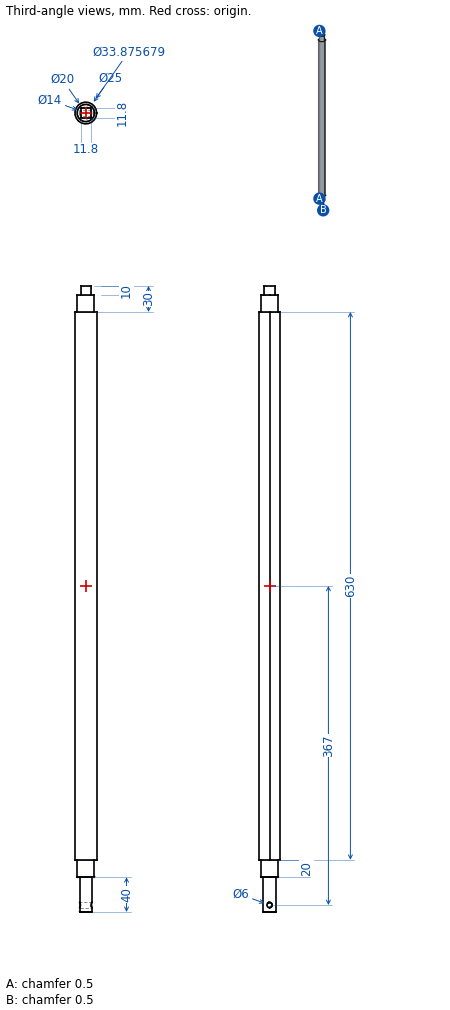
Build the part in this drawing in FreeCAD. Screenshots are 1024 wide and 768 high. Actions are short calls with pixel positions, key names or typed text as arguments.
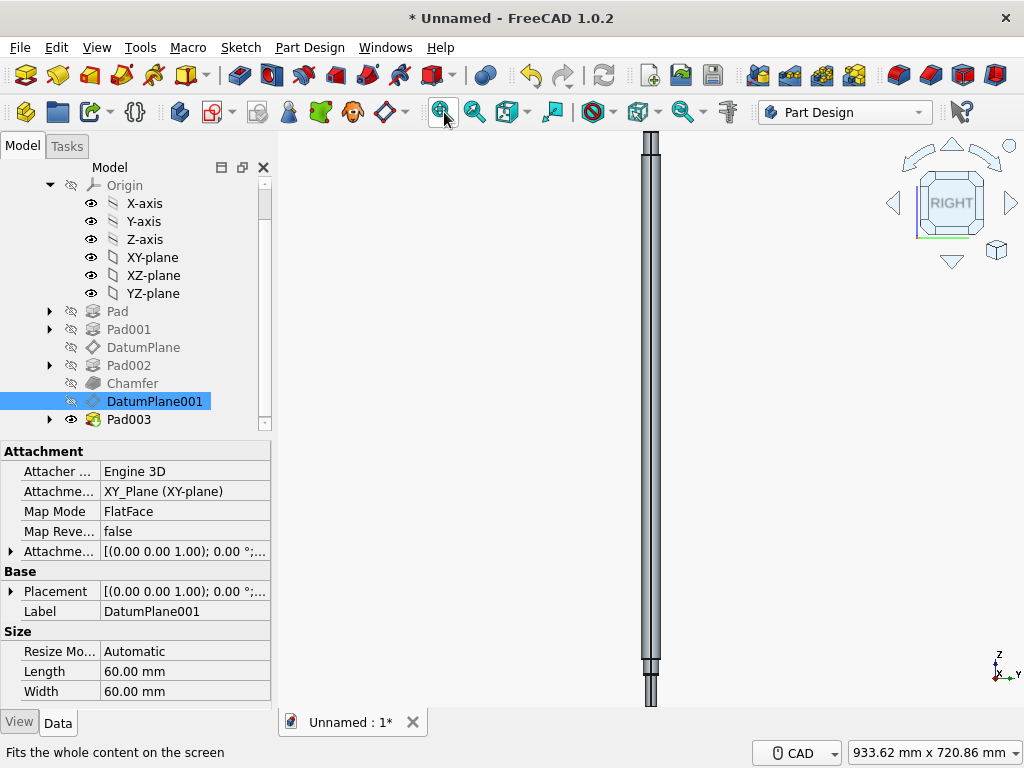
key(0)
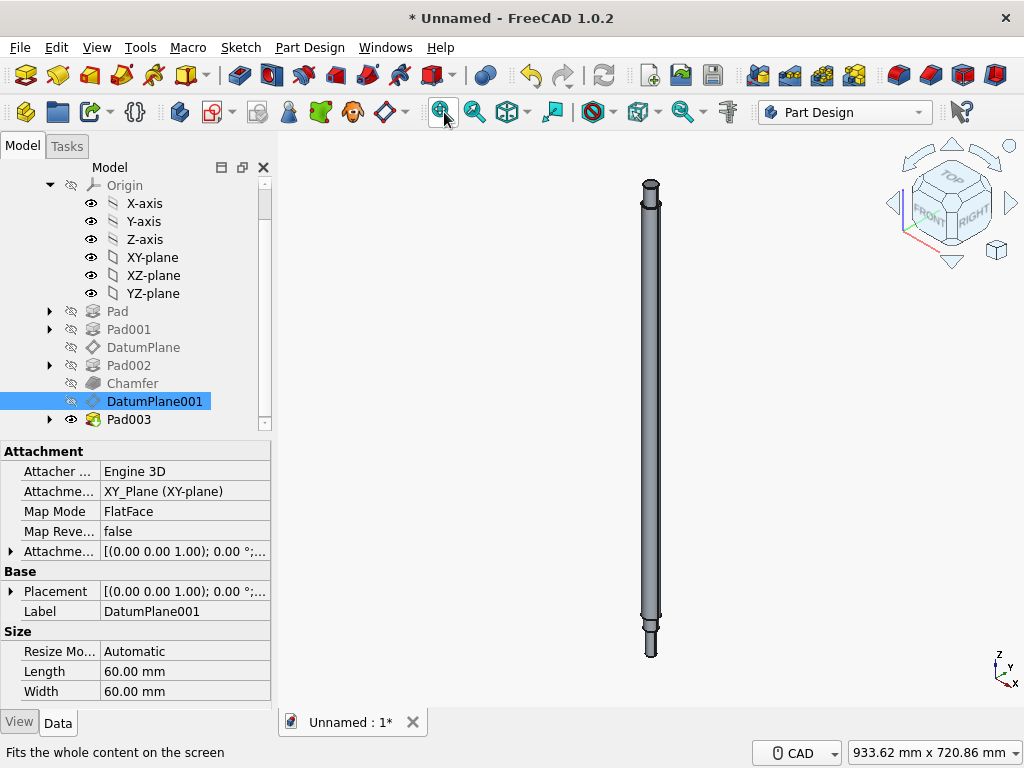
click(656, 655)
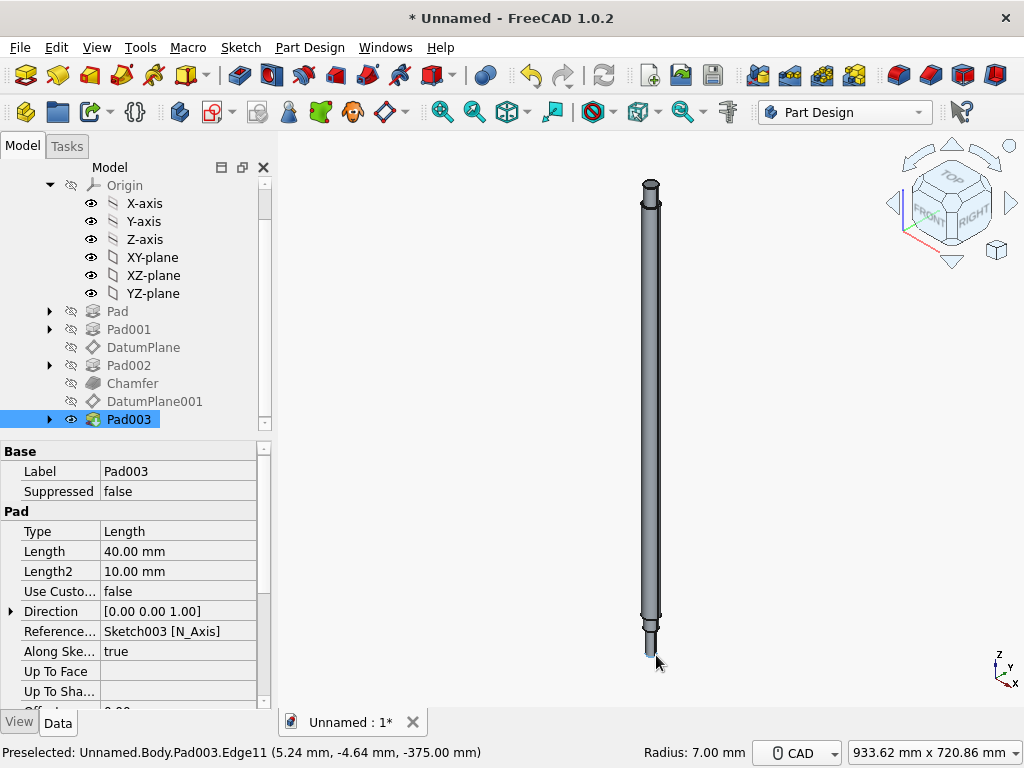
click(932, 76)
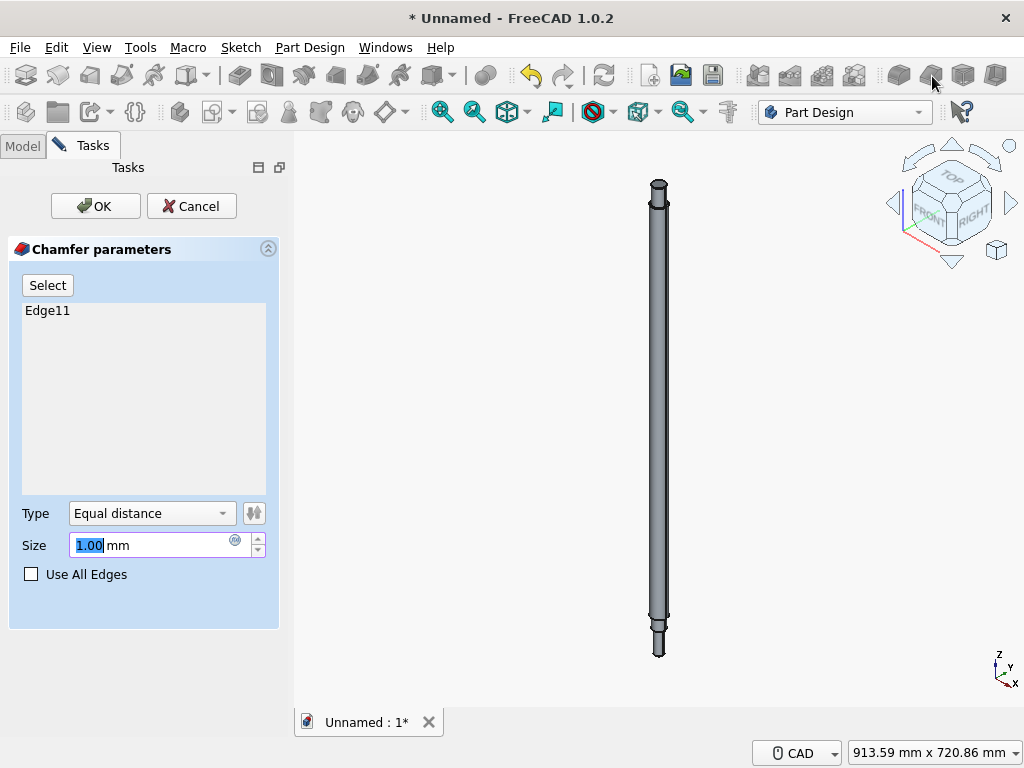
text(0.5)
key(Tab)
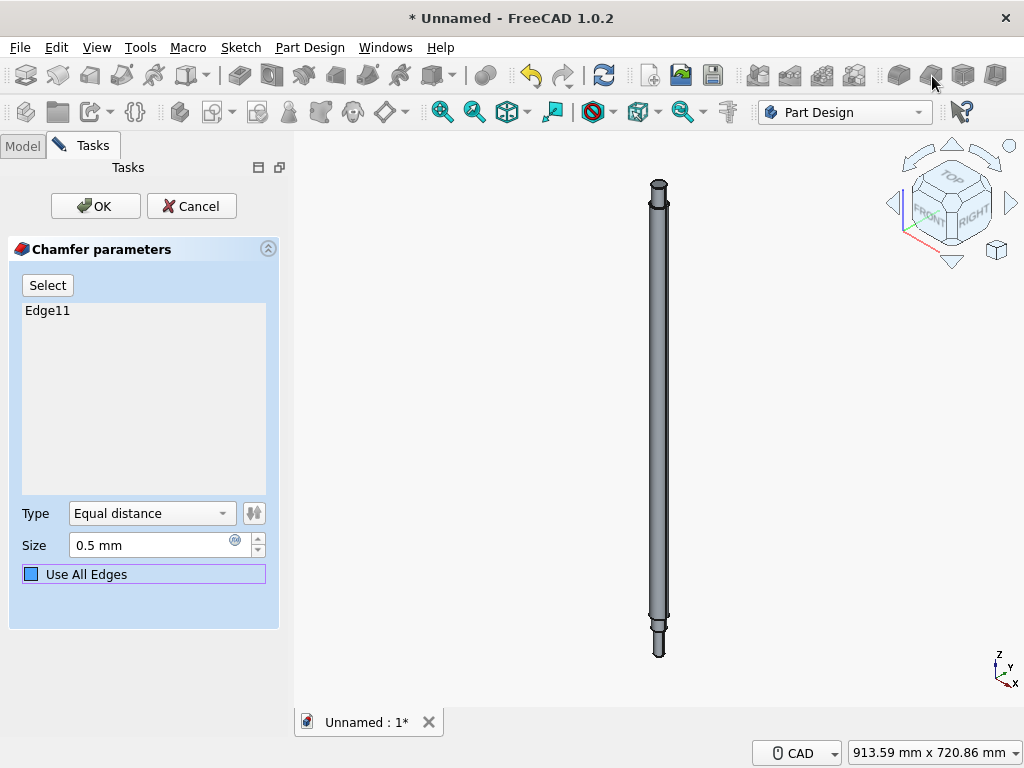
click(96, 206)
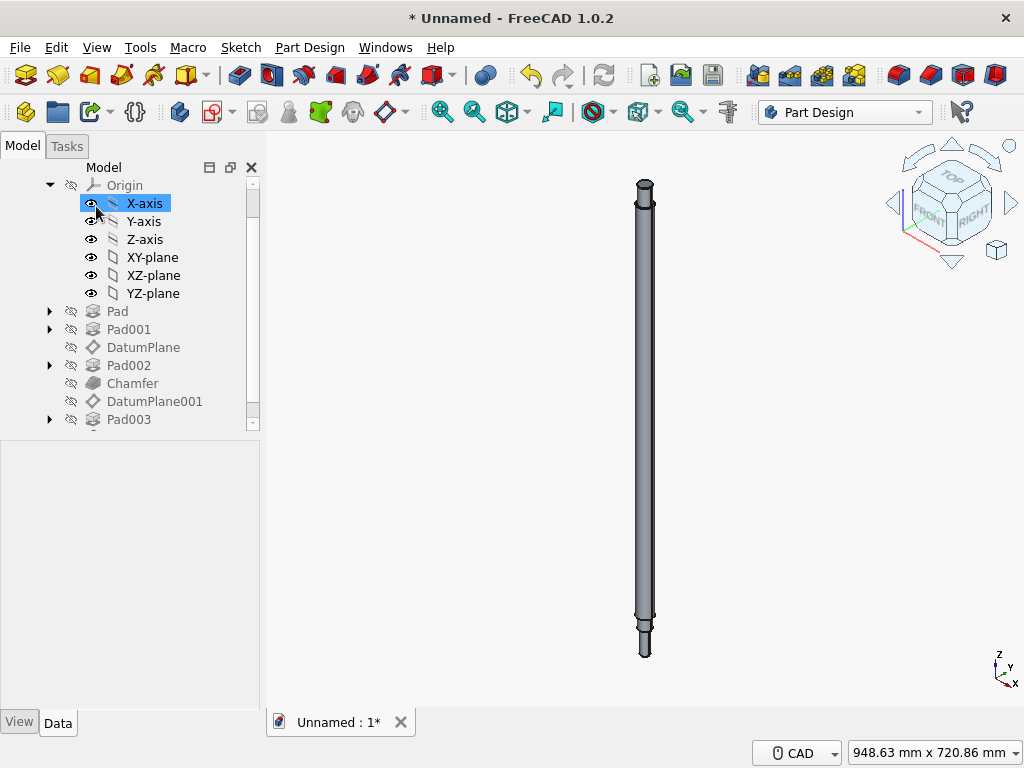
click(212, 112)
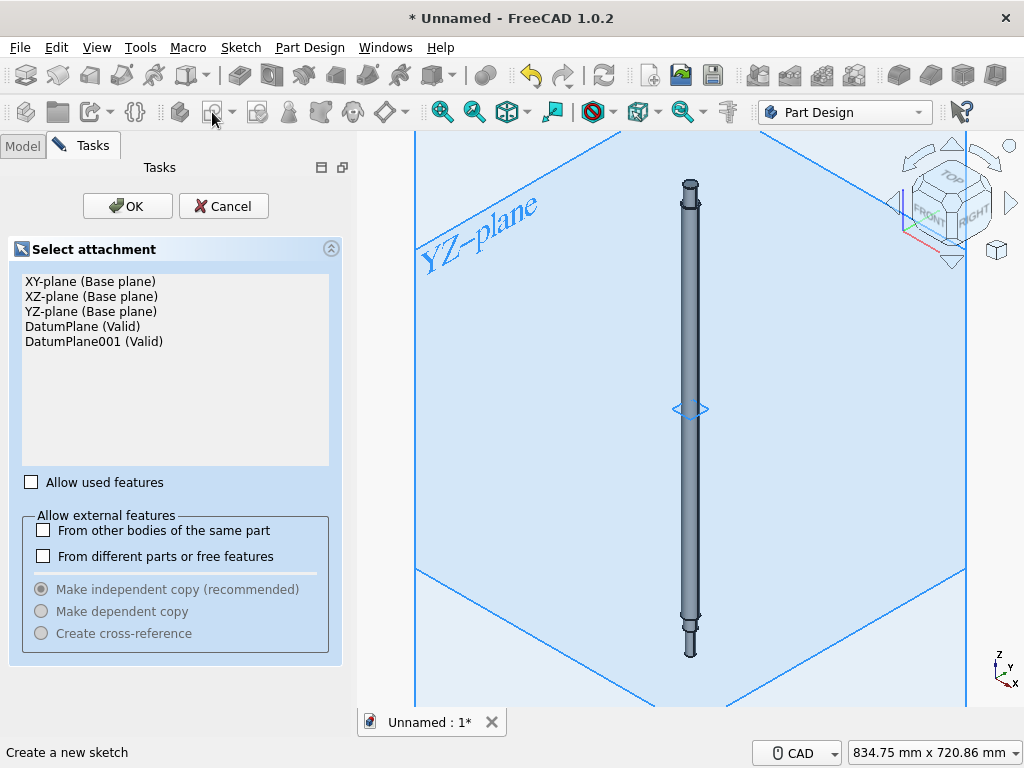
click(82, 312)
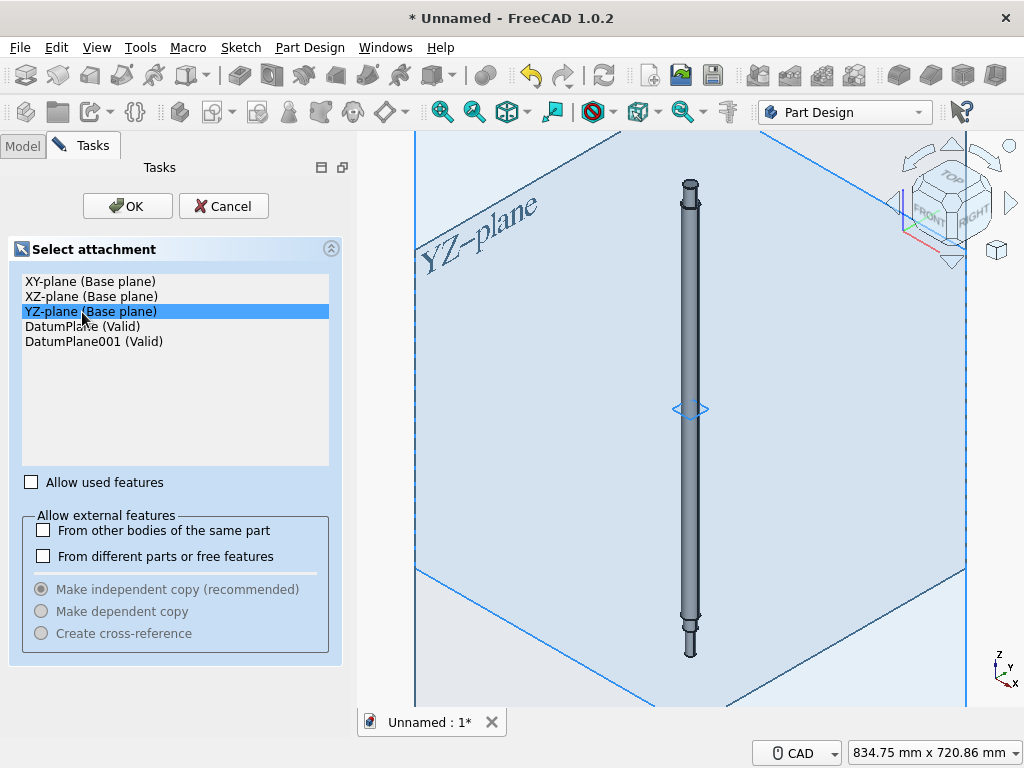
click(128, 206)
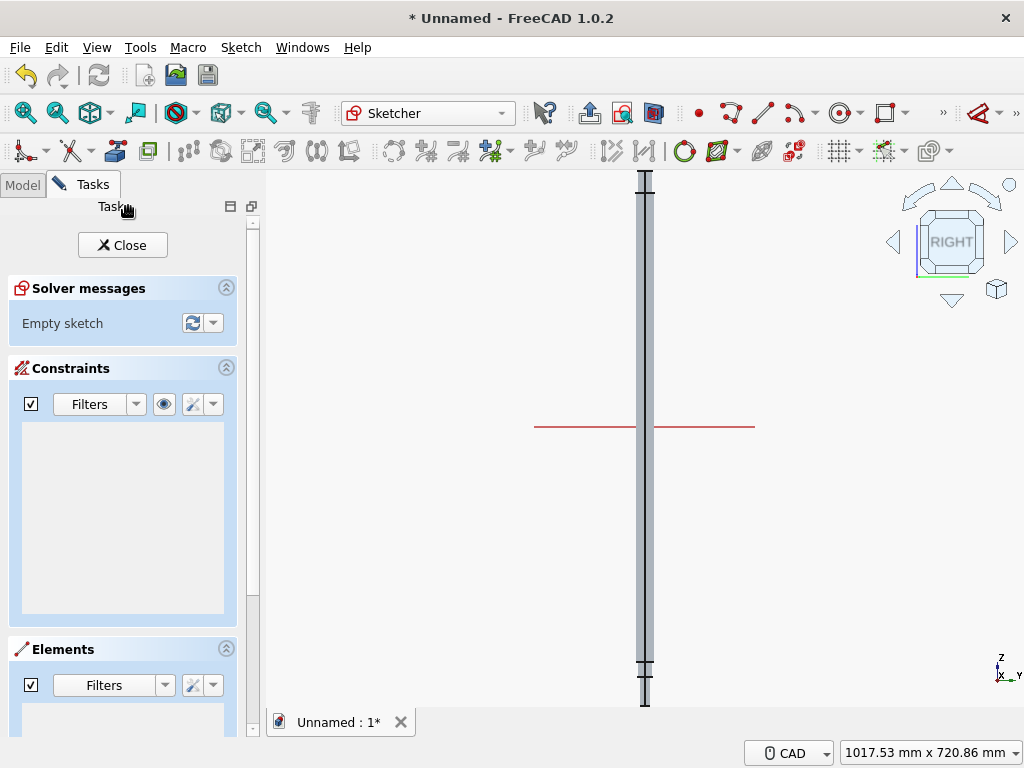
click(654, 114)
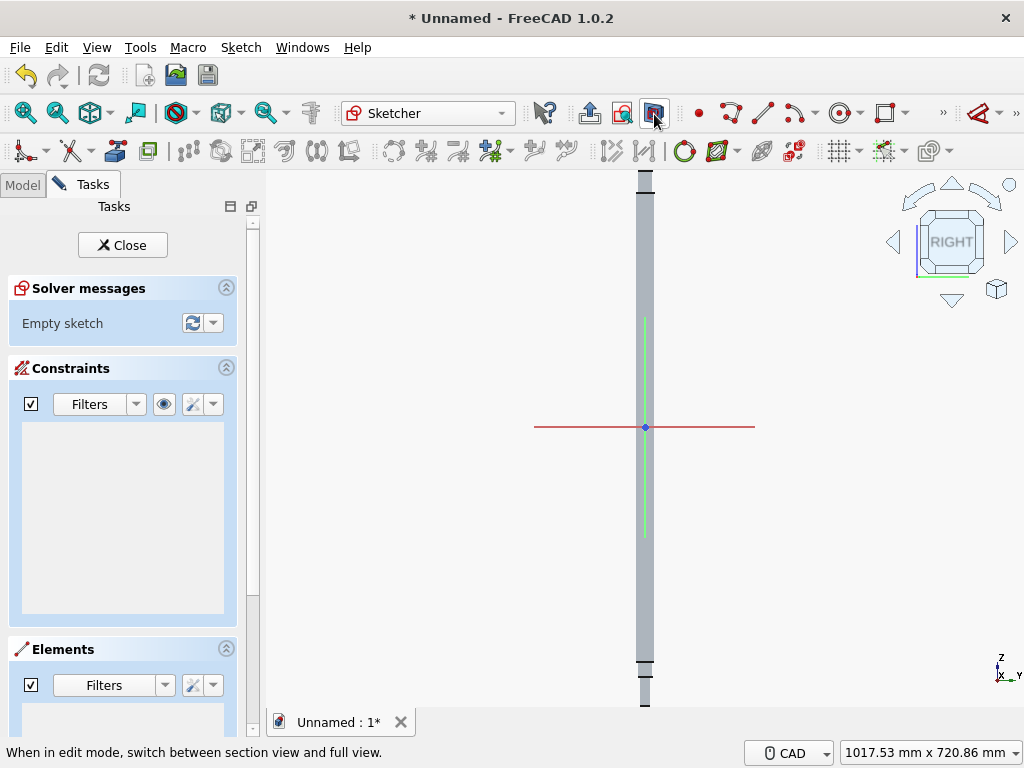
scroll(576, 438, down, 5)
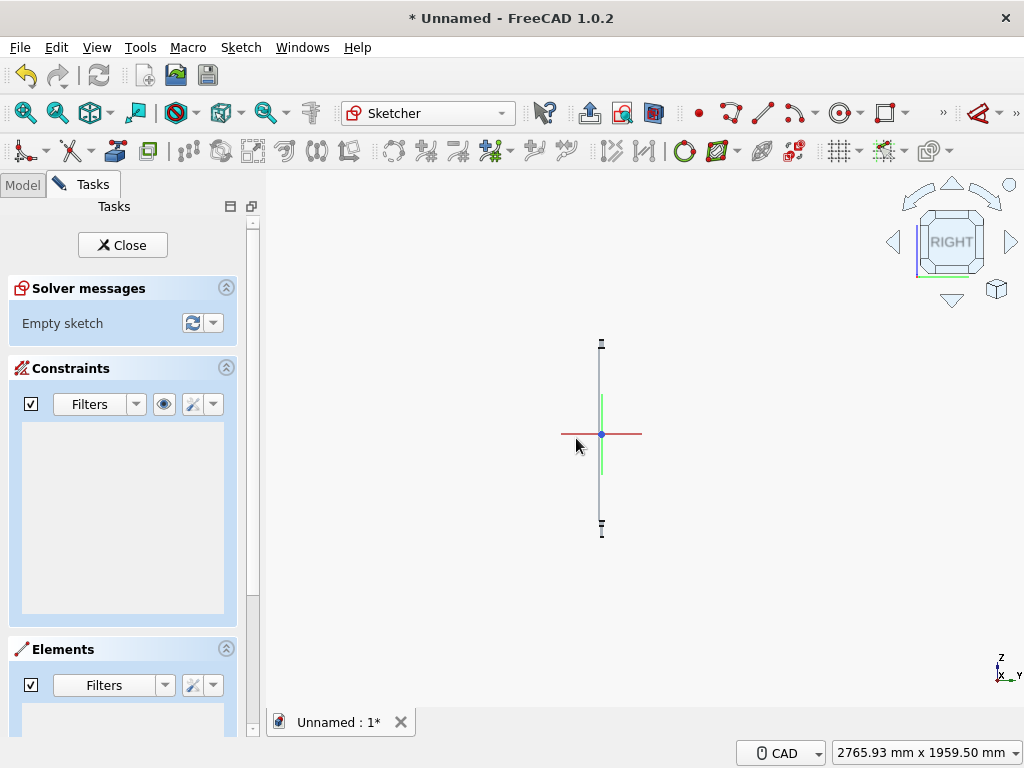
scroll(603, 540, up, 15)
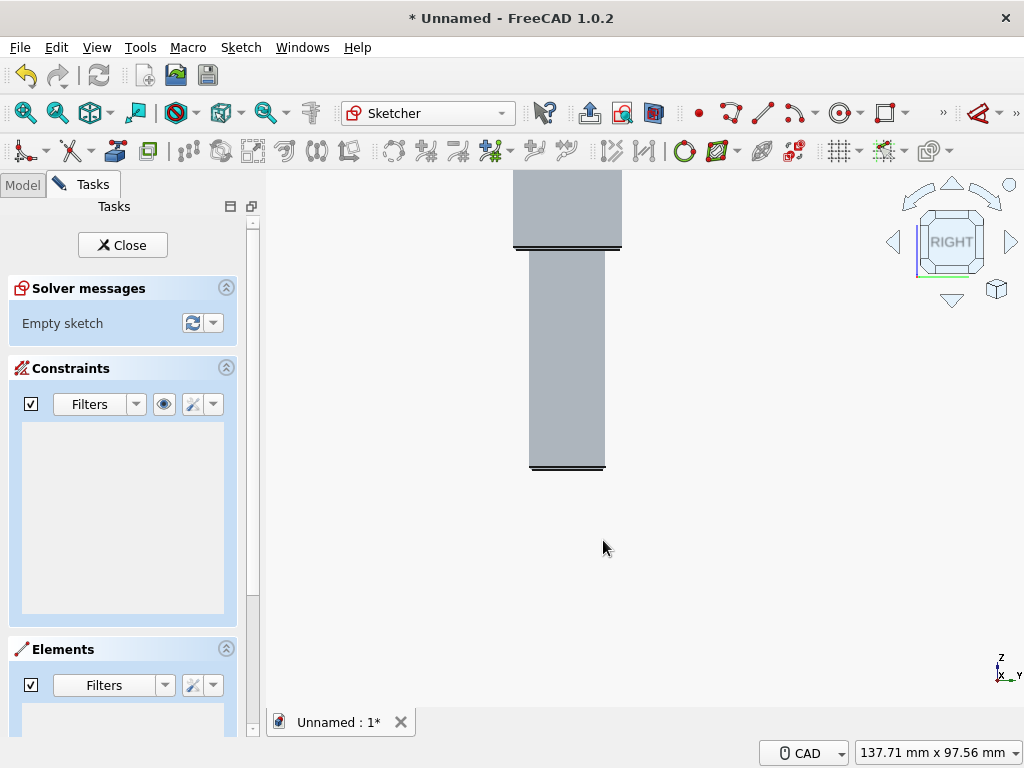
scroll(566, 424, up, 12)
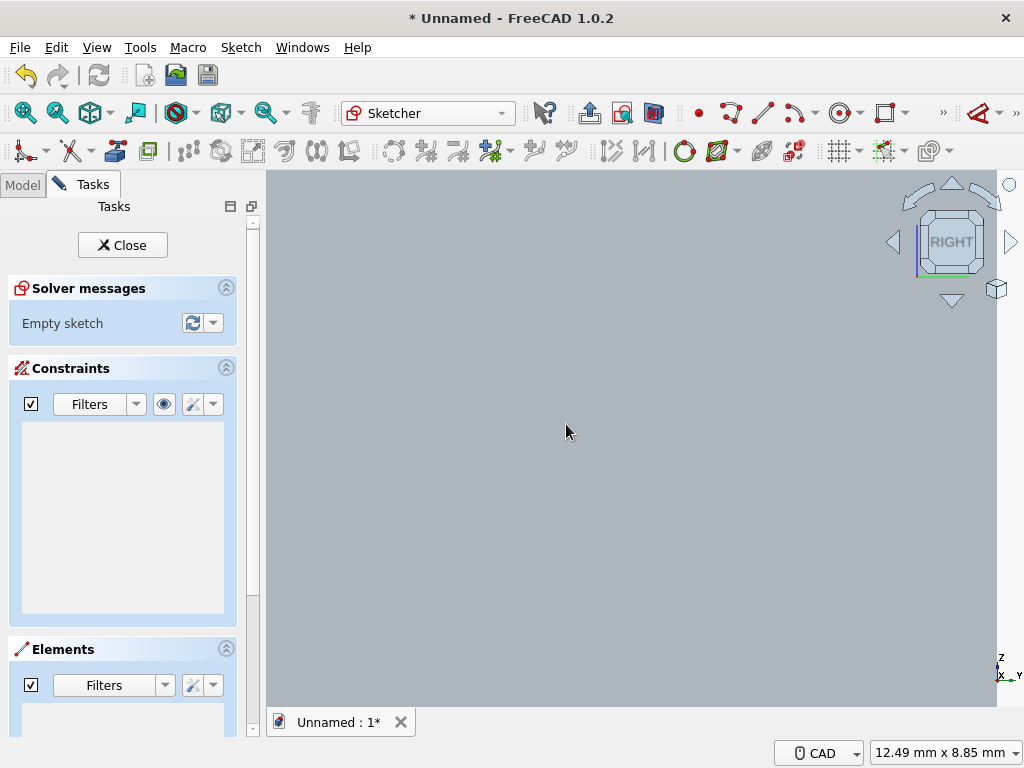
click(840, 114)